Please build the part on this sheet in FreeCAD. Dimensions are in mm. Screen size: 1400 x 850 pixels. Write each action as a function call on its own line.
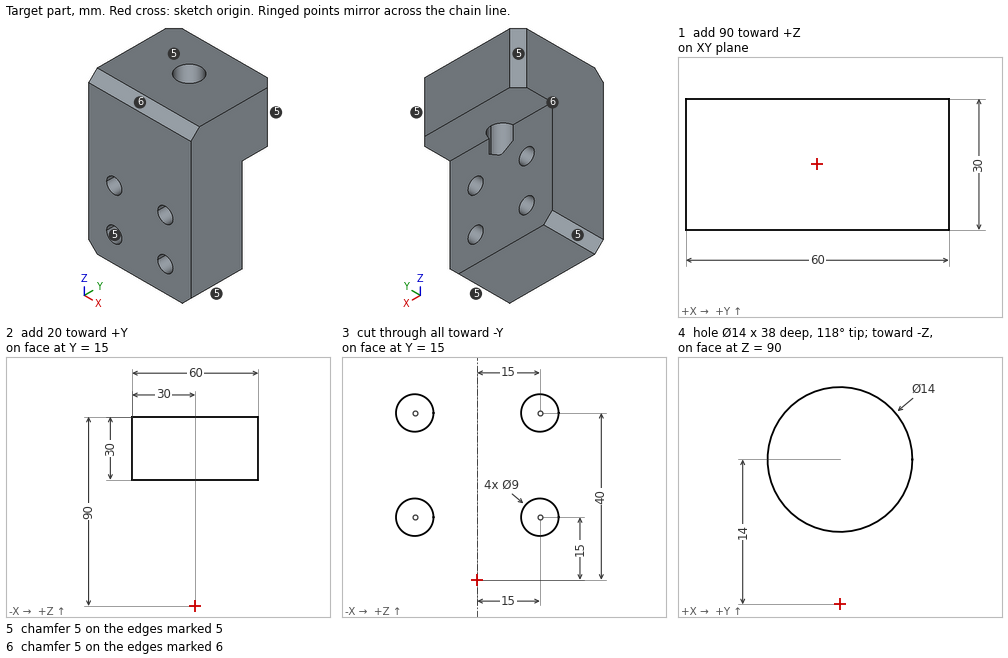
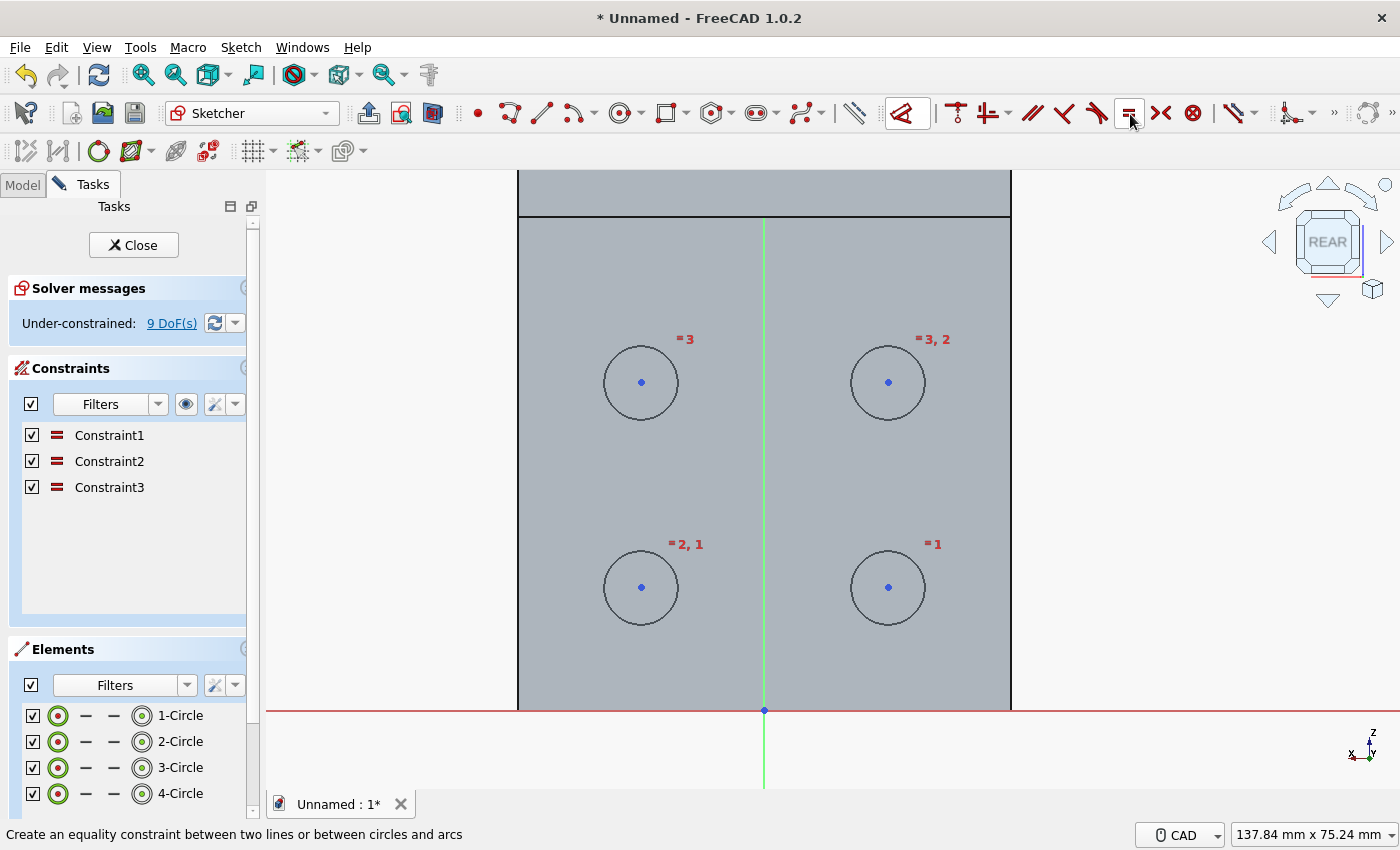
click(888, 588)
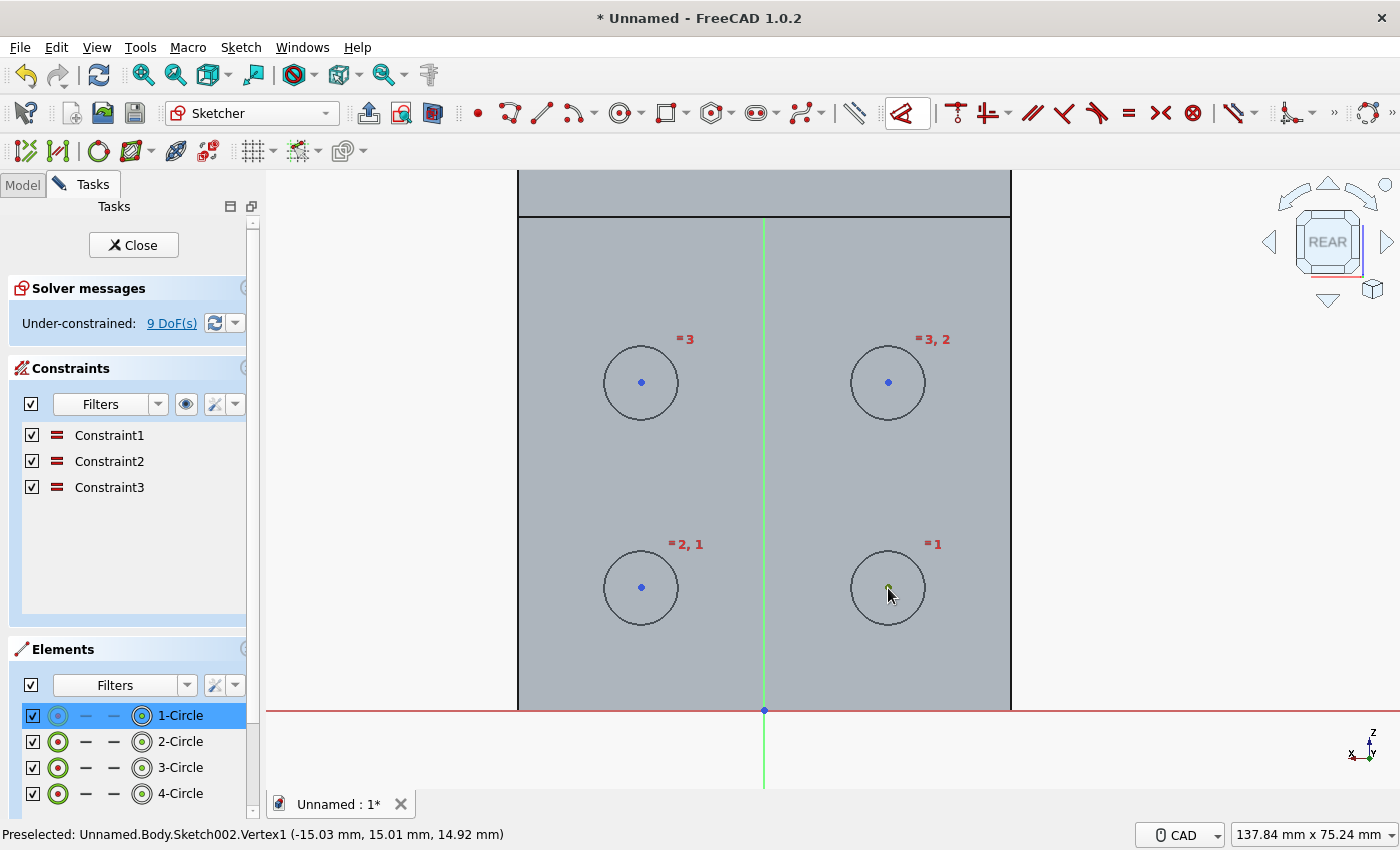
click(641, 588)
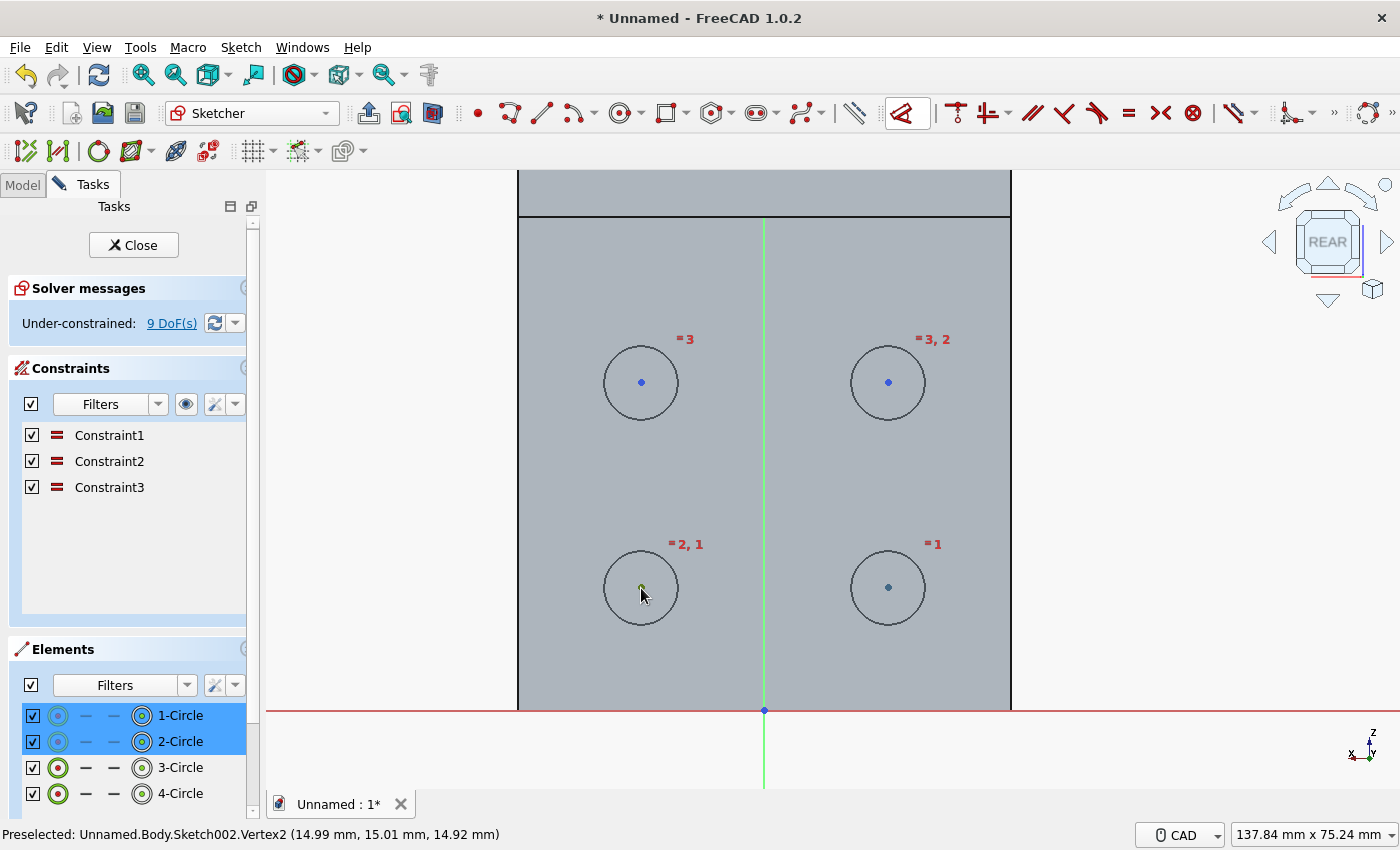
click(764, 681)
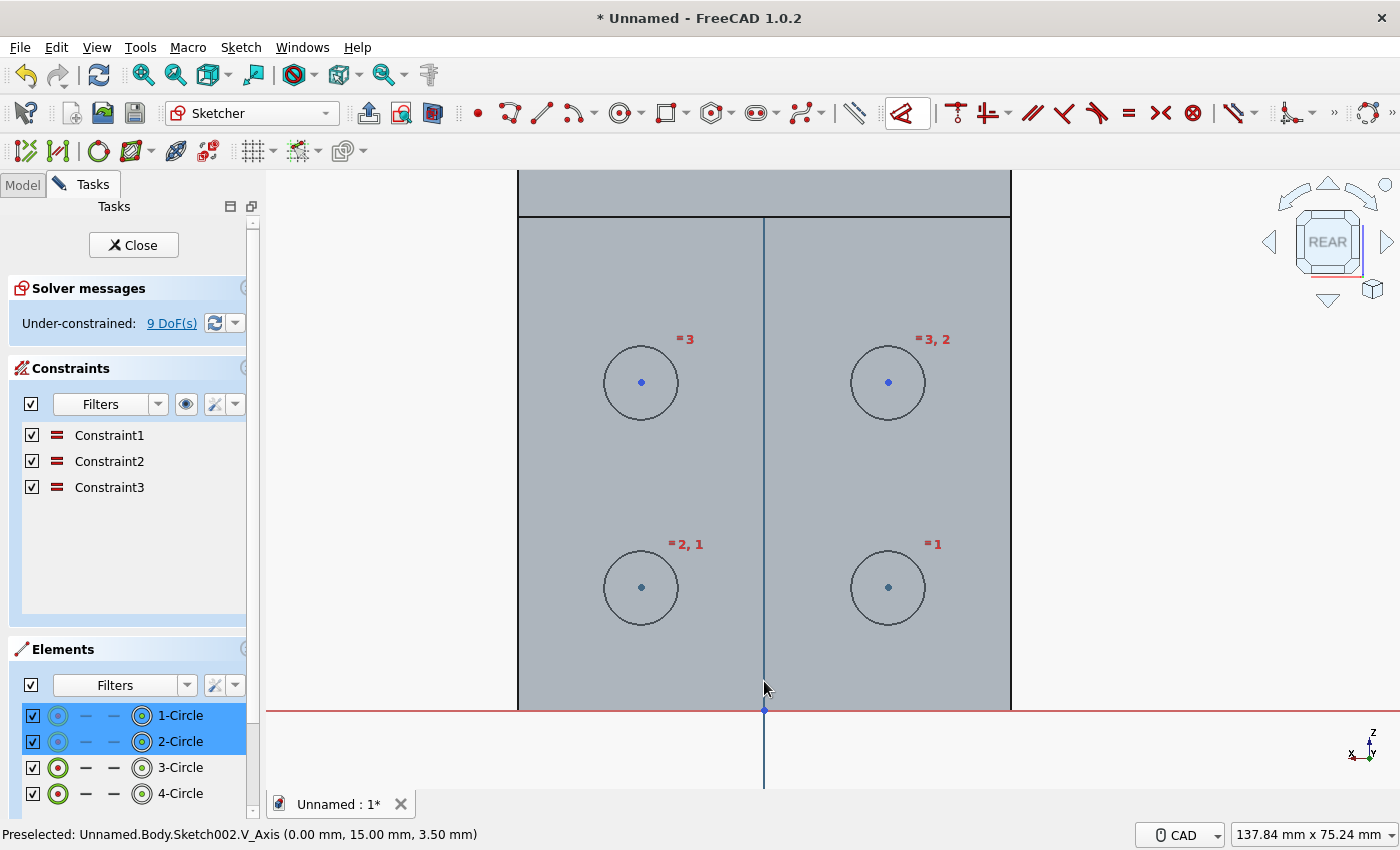
key(s)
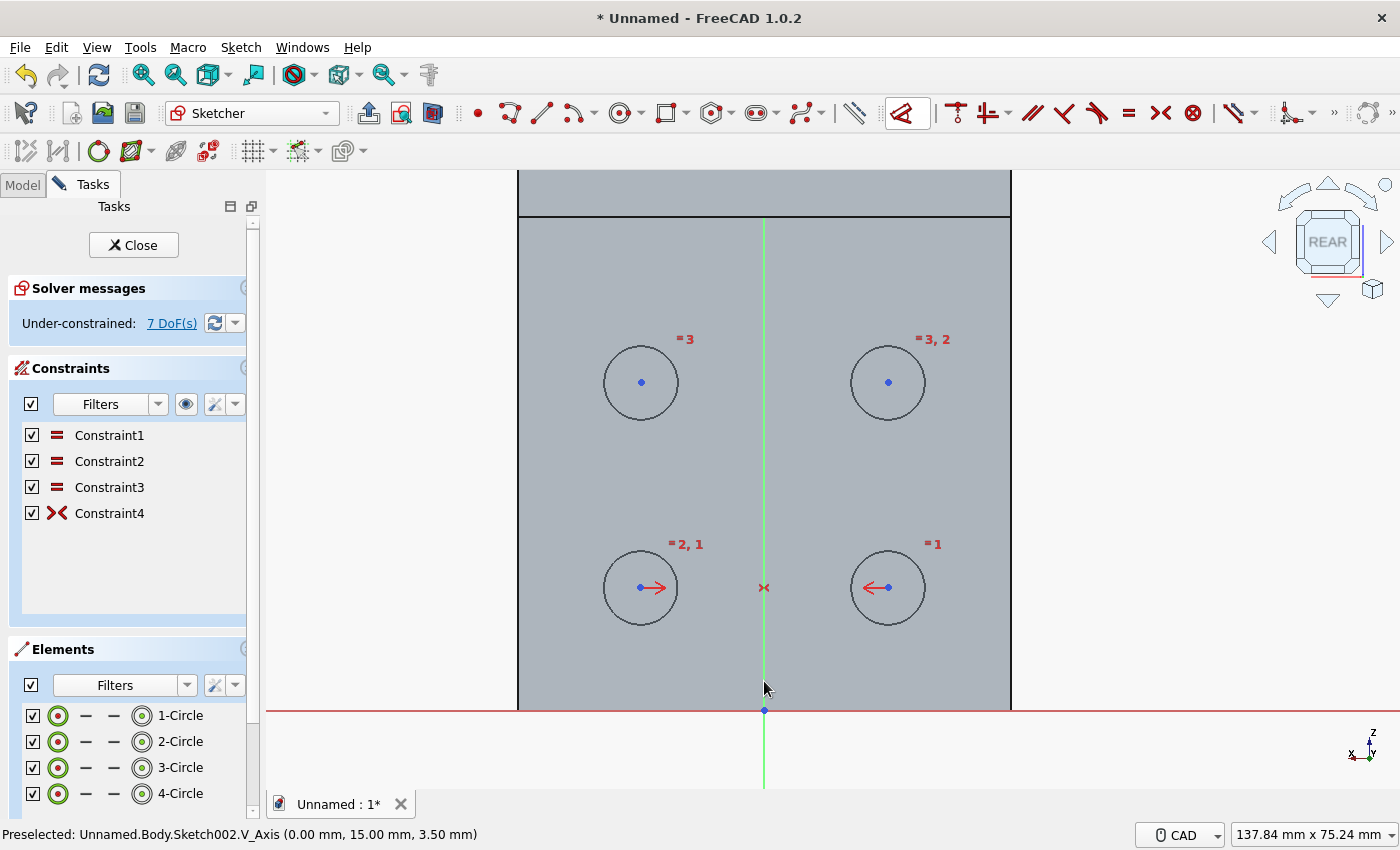
click(888, 383)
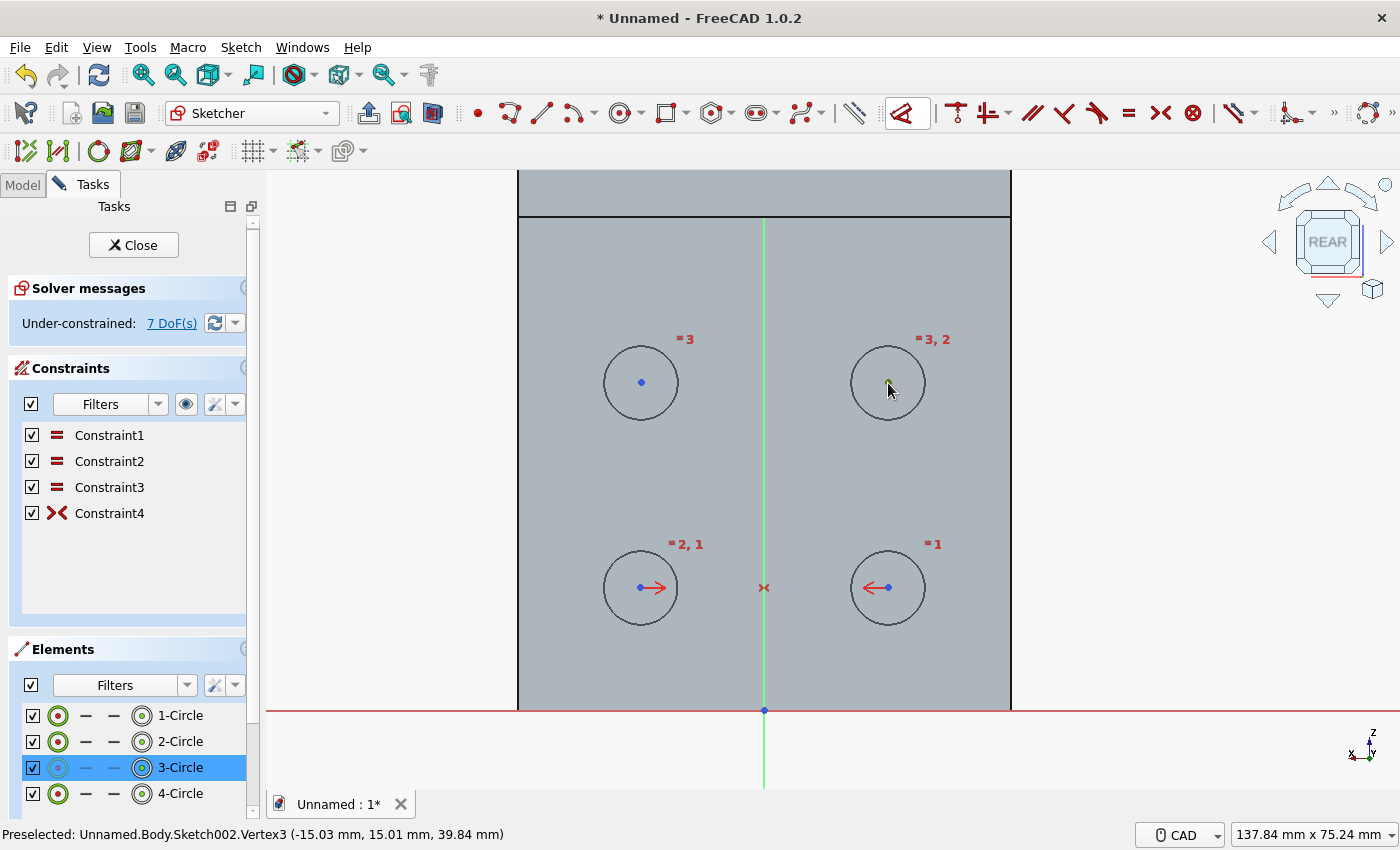
click(641, 383)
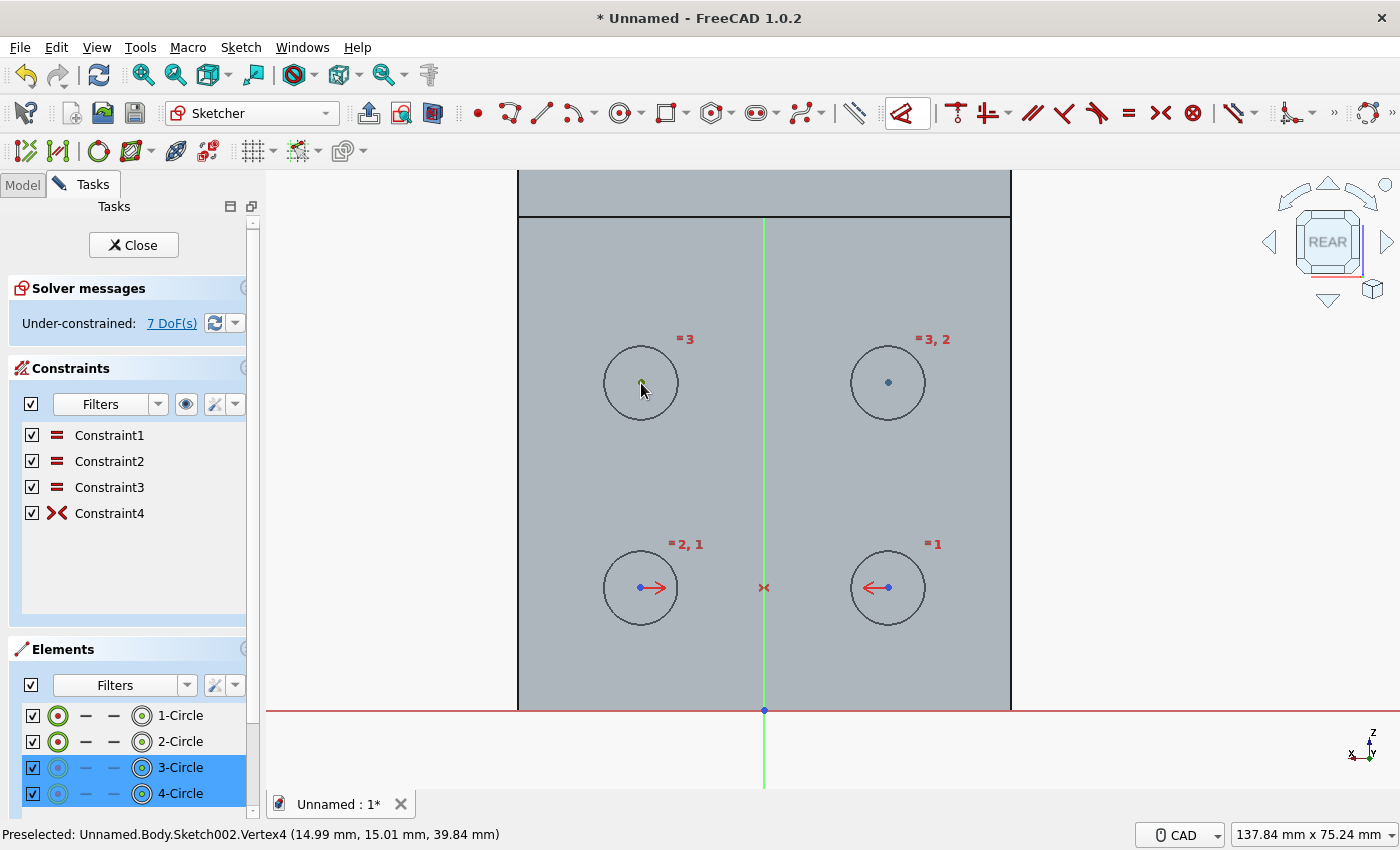
click(764, 681)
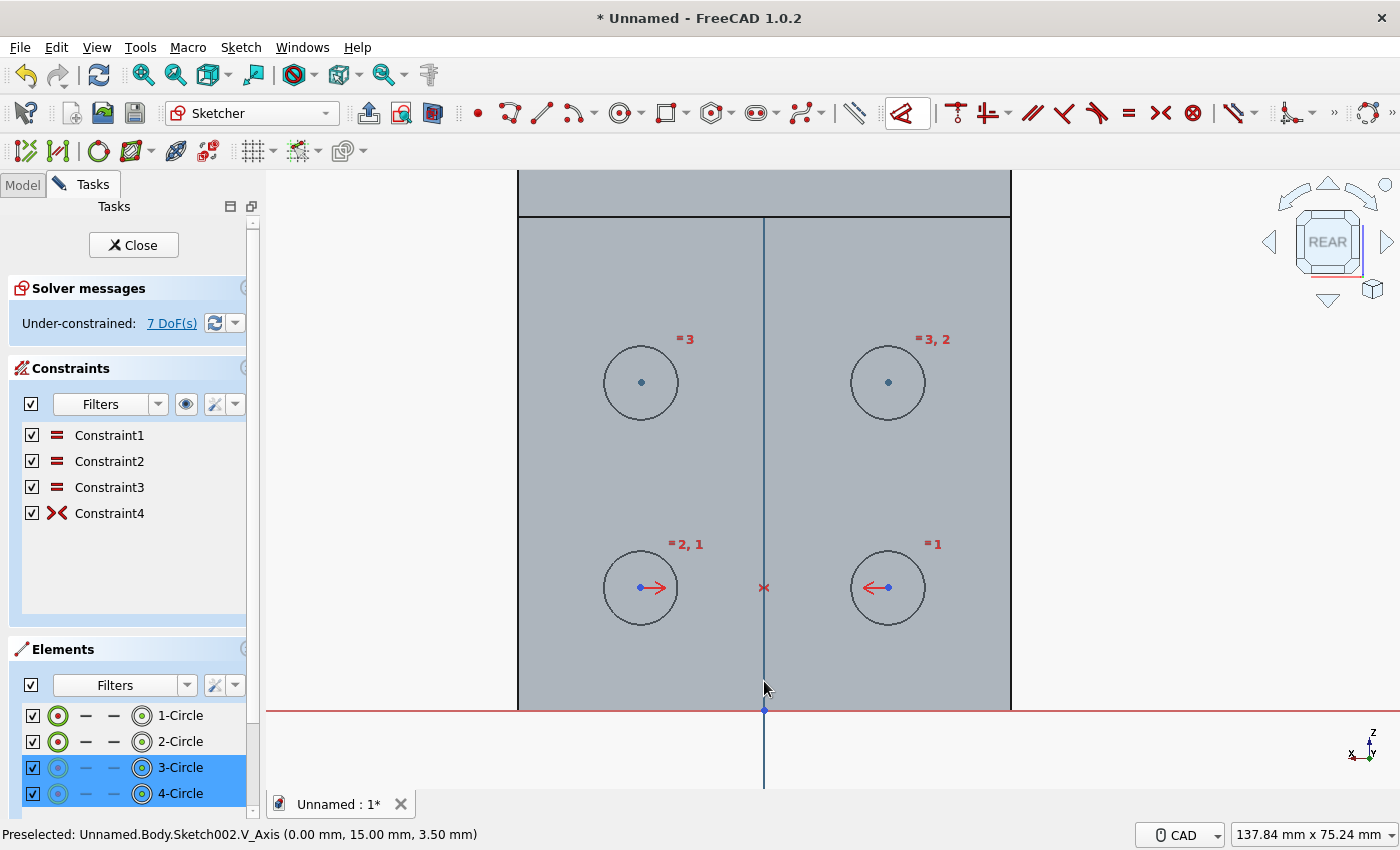
click(1162, 114)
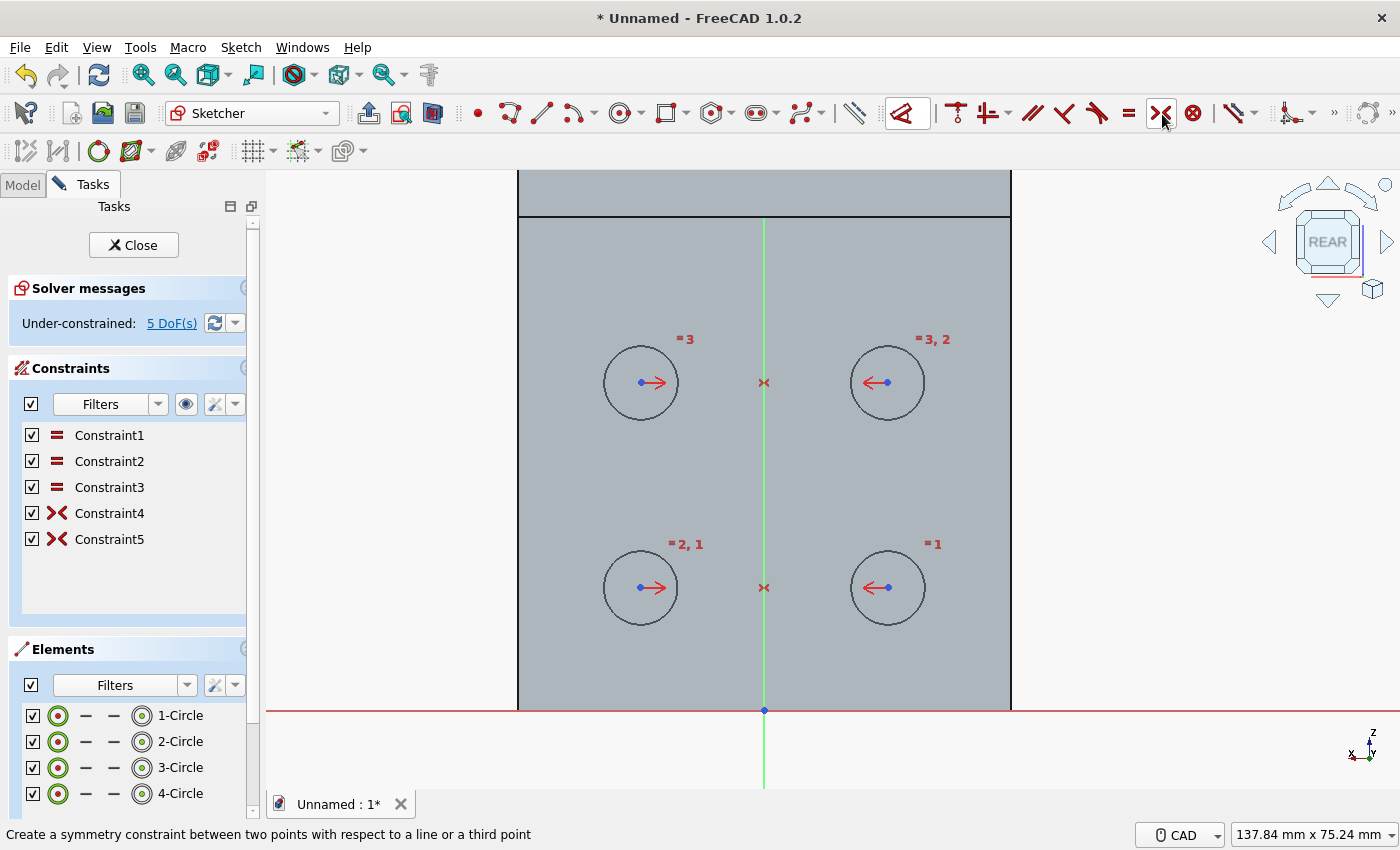
click(914, 562)